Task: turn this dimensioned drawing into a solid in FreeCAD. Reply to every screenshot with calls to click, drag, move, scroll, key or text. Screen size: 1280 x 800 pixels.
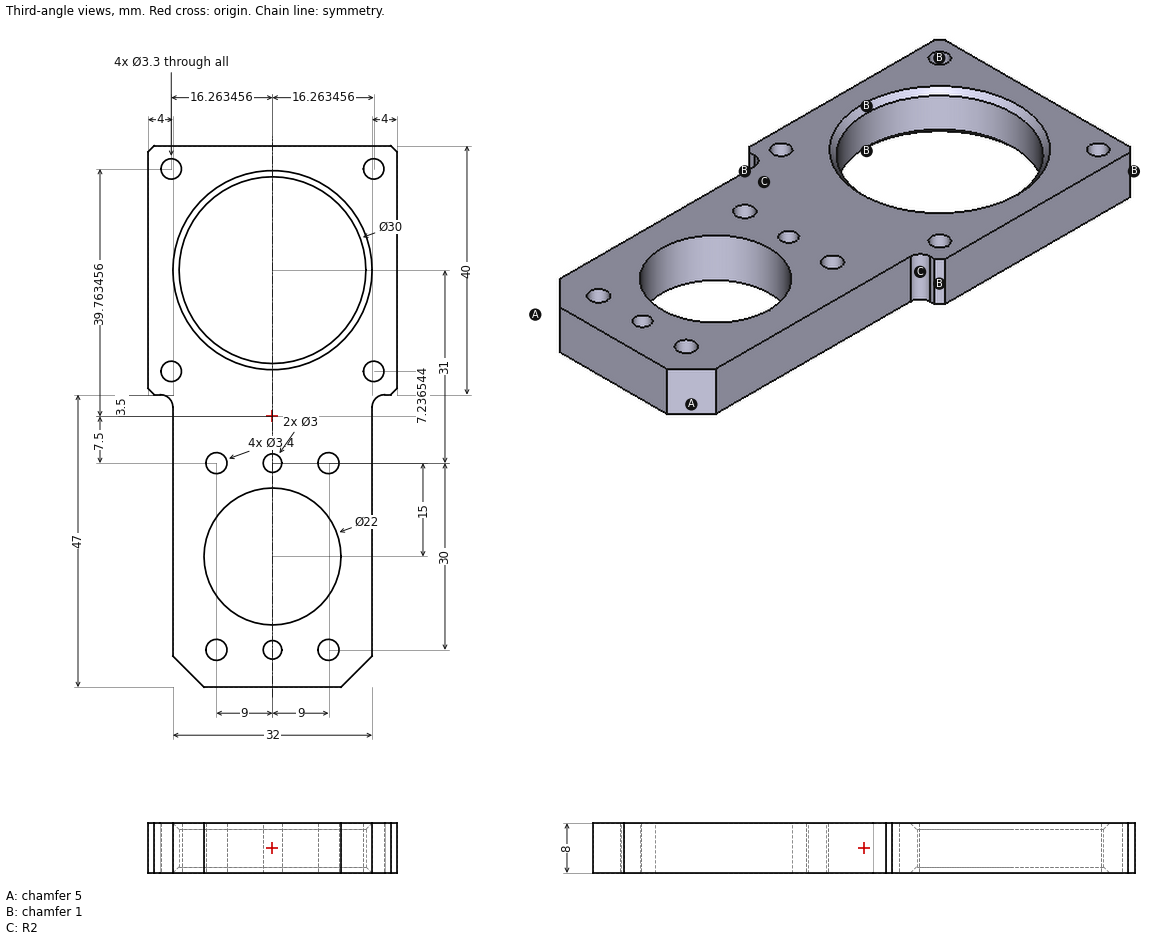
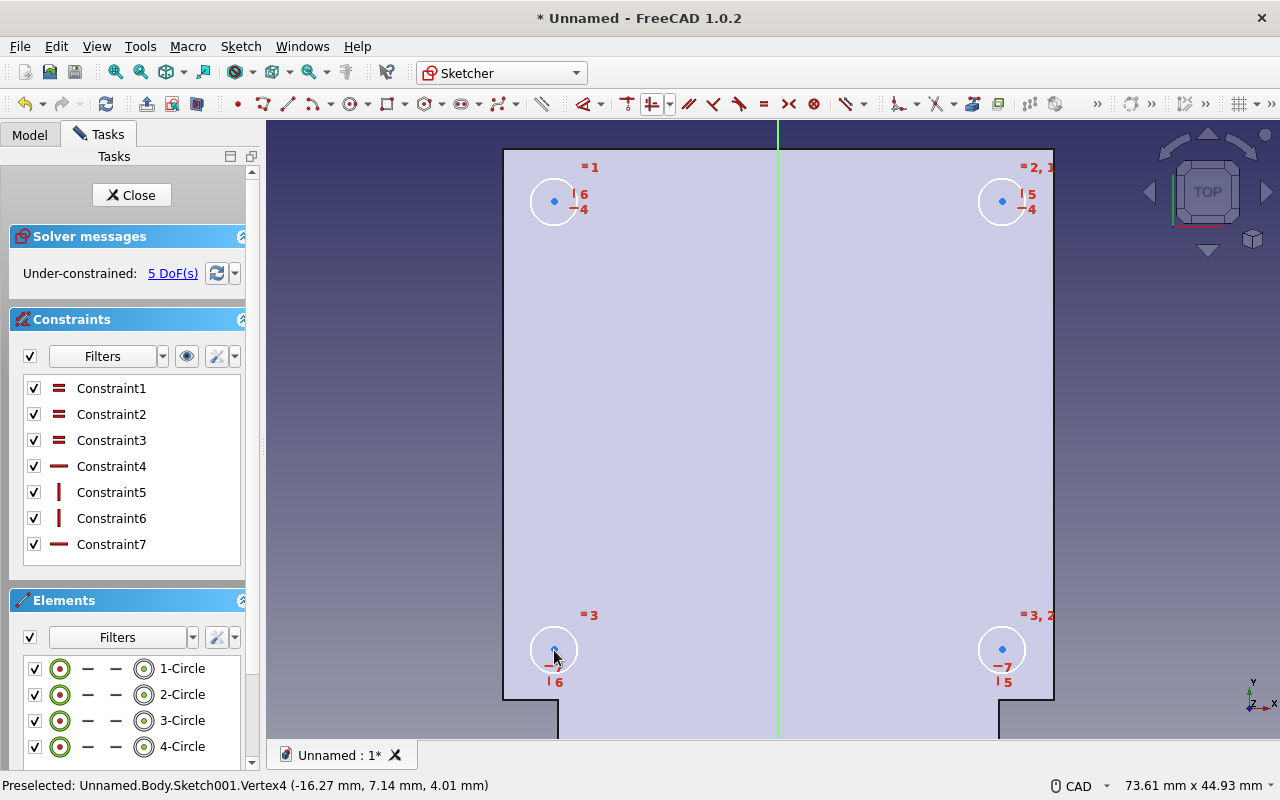
click(582, 104)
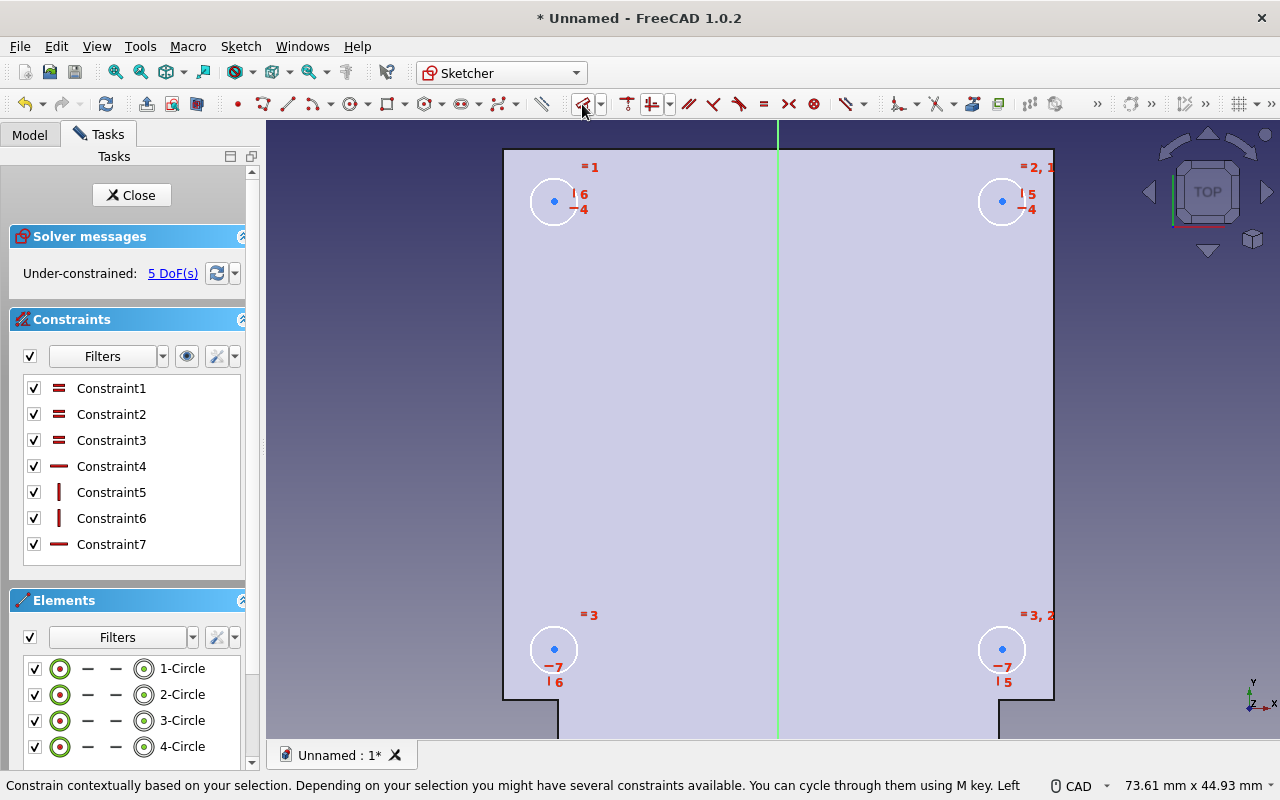
click(570, 185)
click(592, 162)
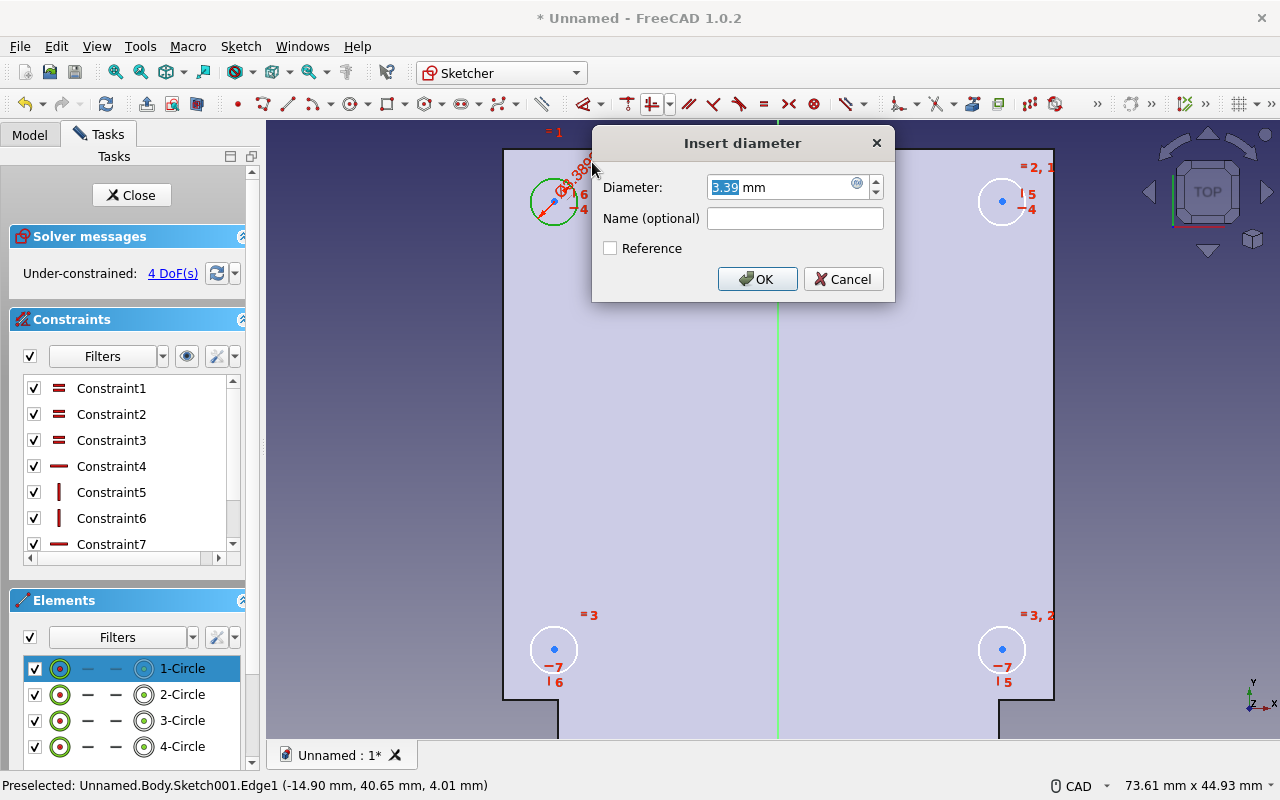
text(3.3)
key(Return)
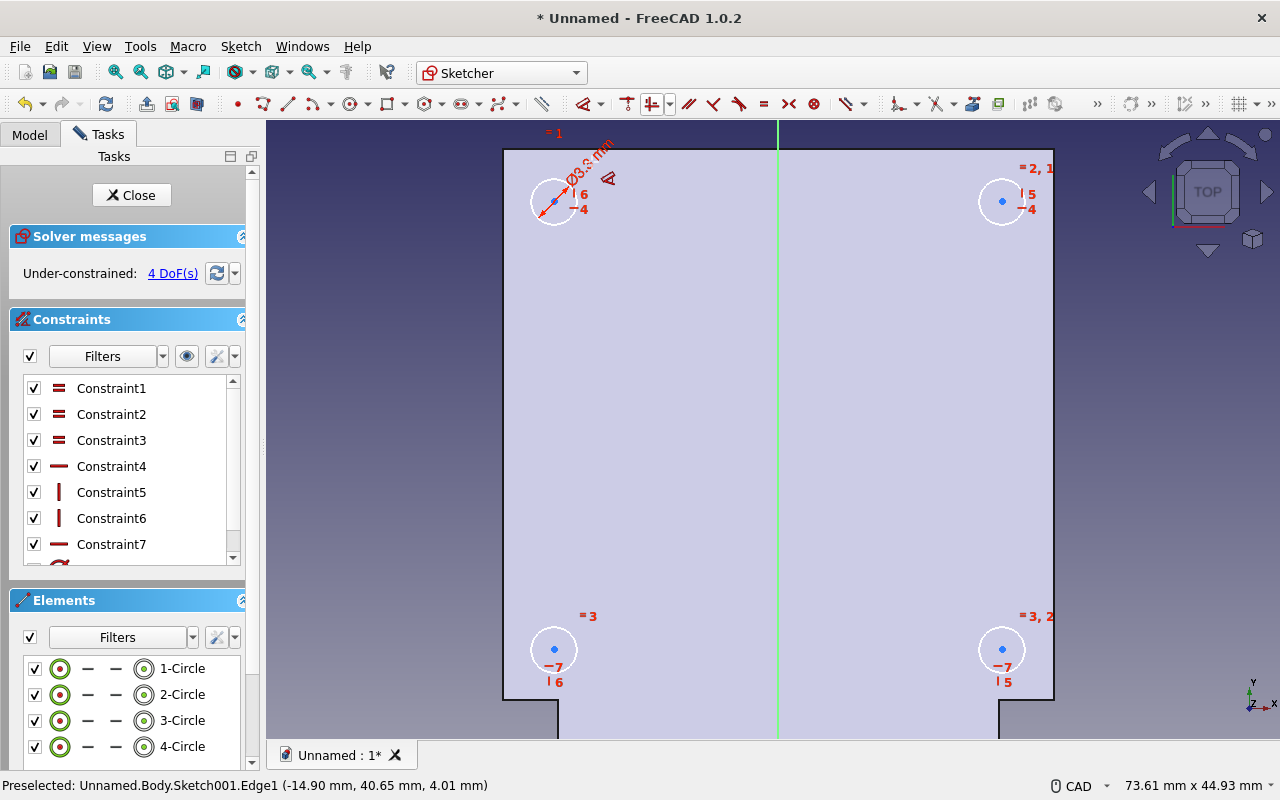
click(1002, 650)
click(1036, 680)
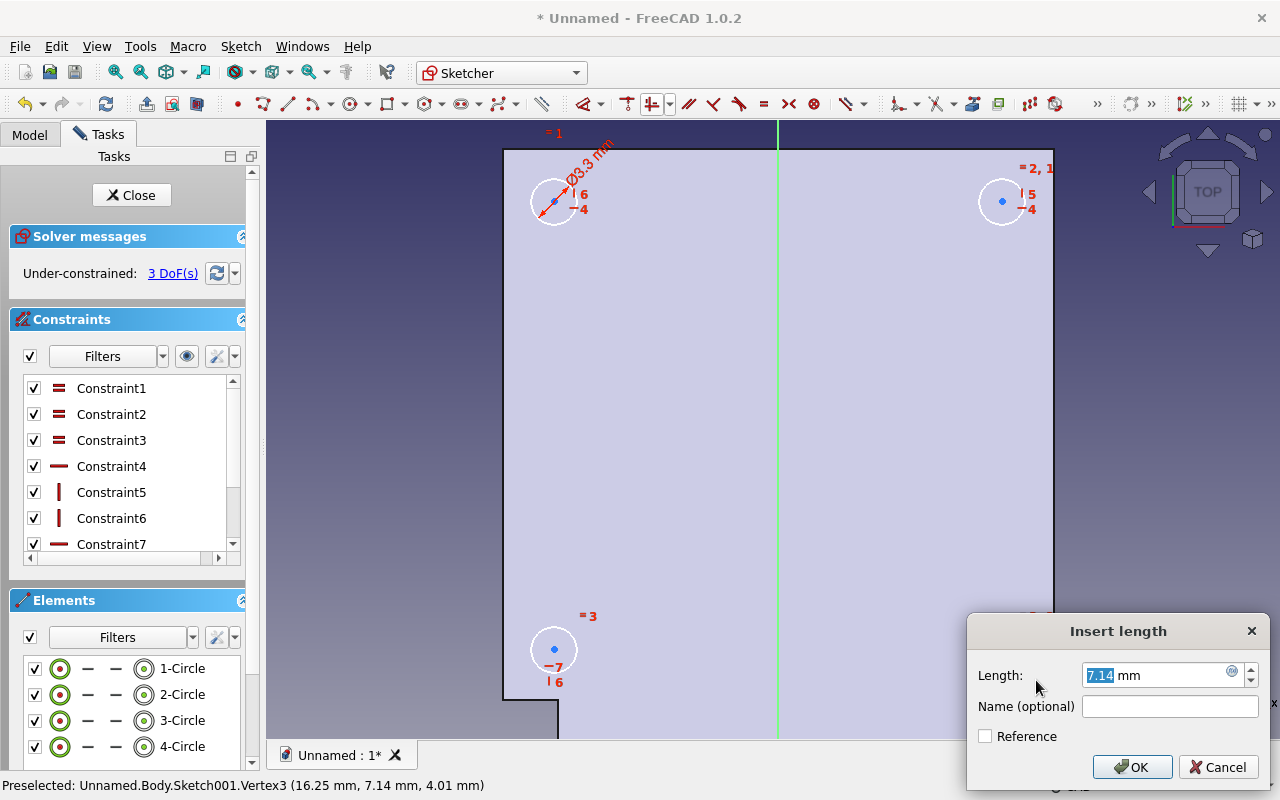
text(7.236544)
key(Return)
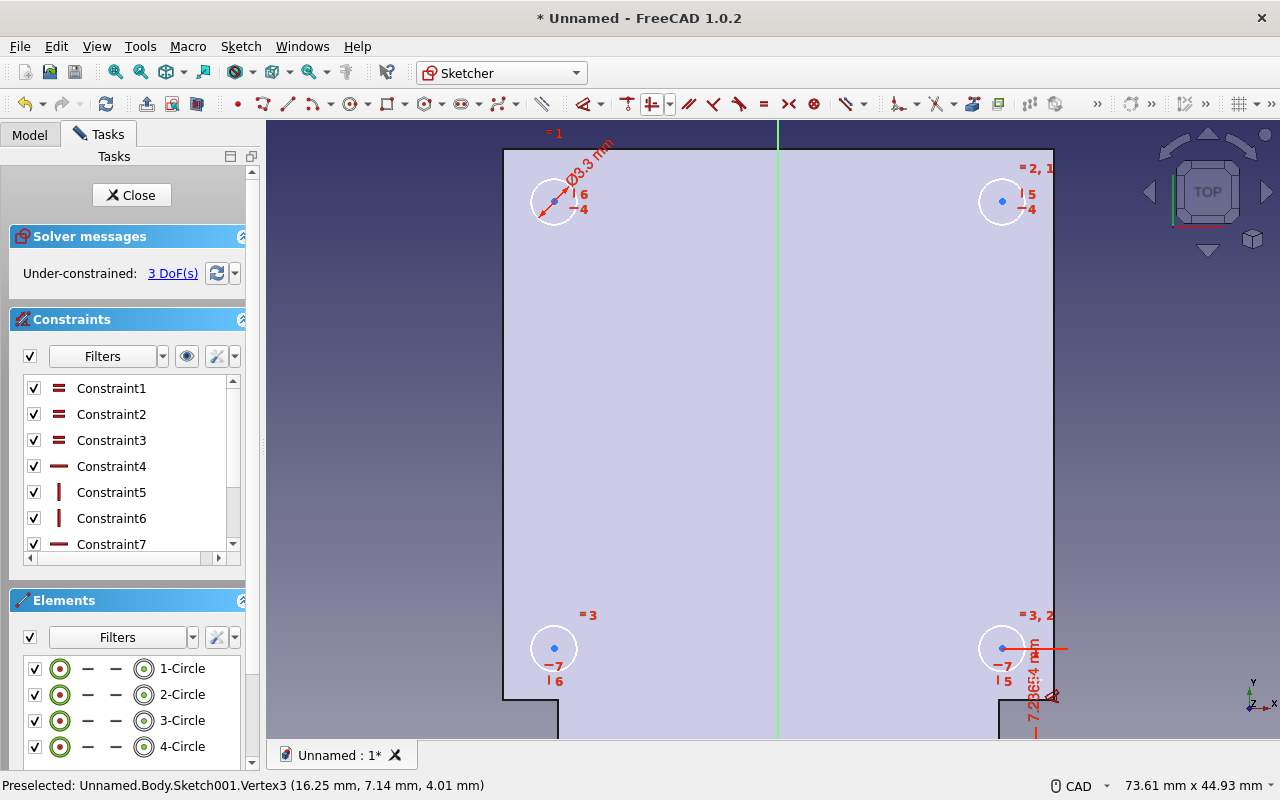
click(554, 202)
click(666, 168)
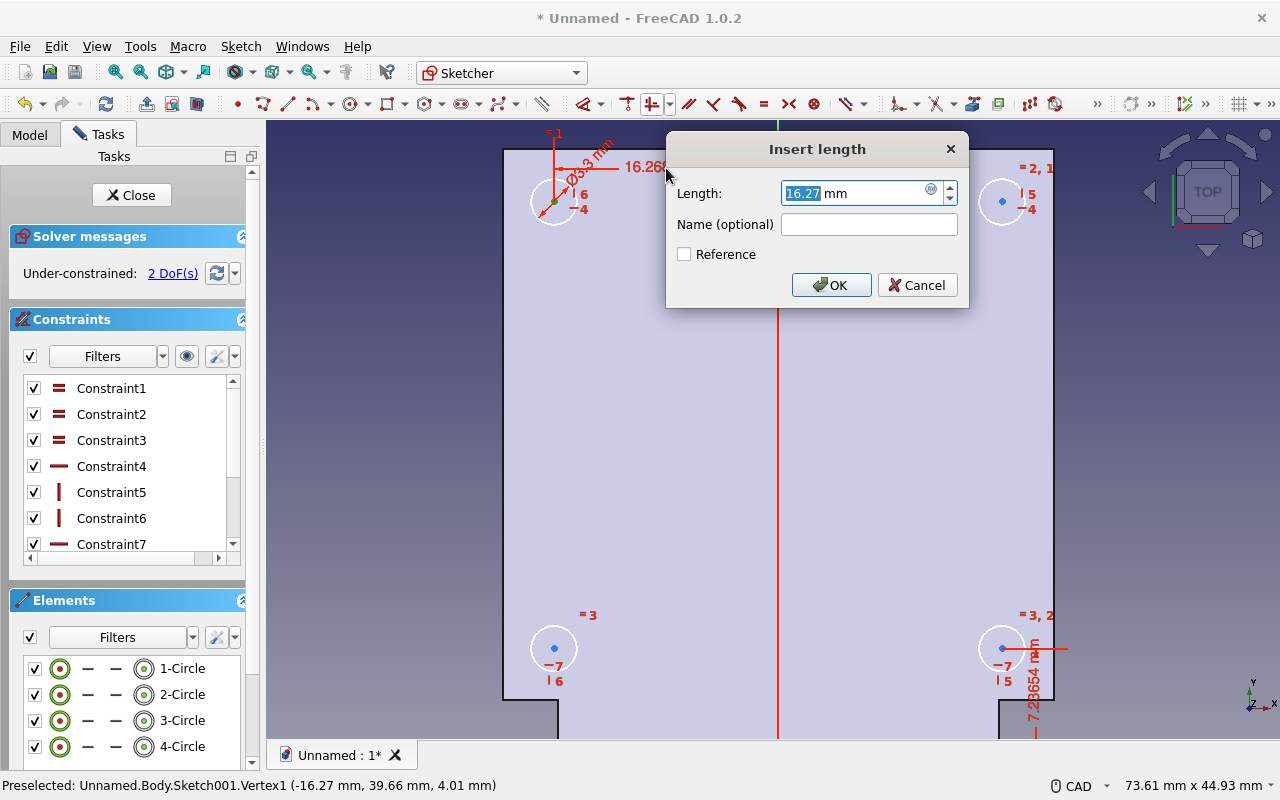
text(16.263456)
key(Return)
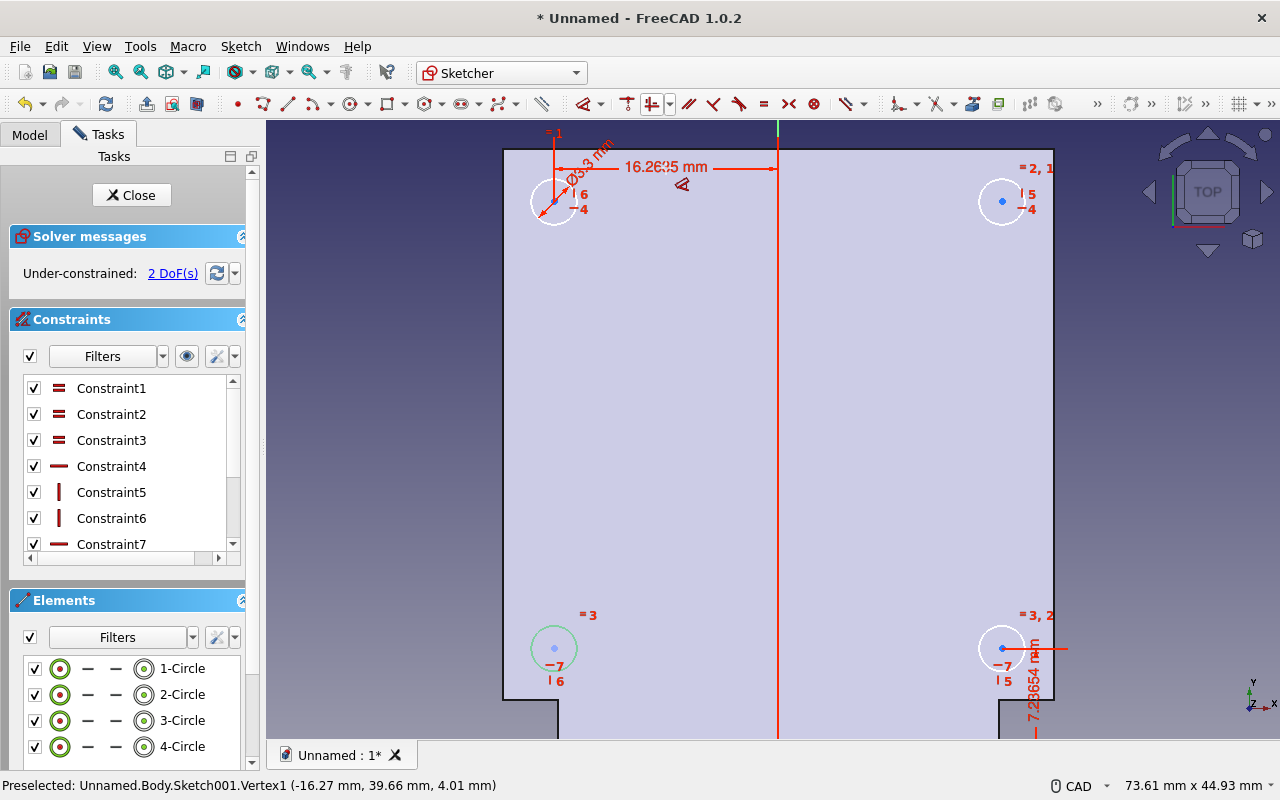
click(554, 202)
click(520, 456)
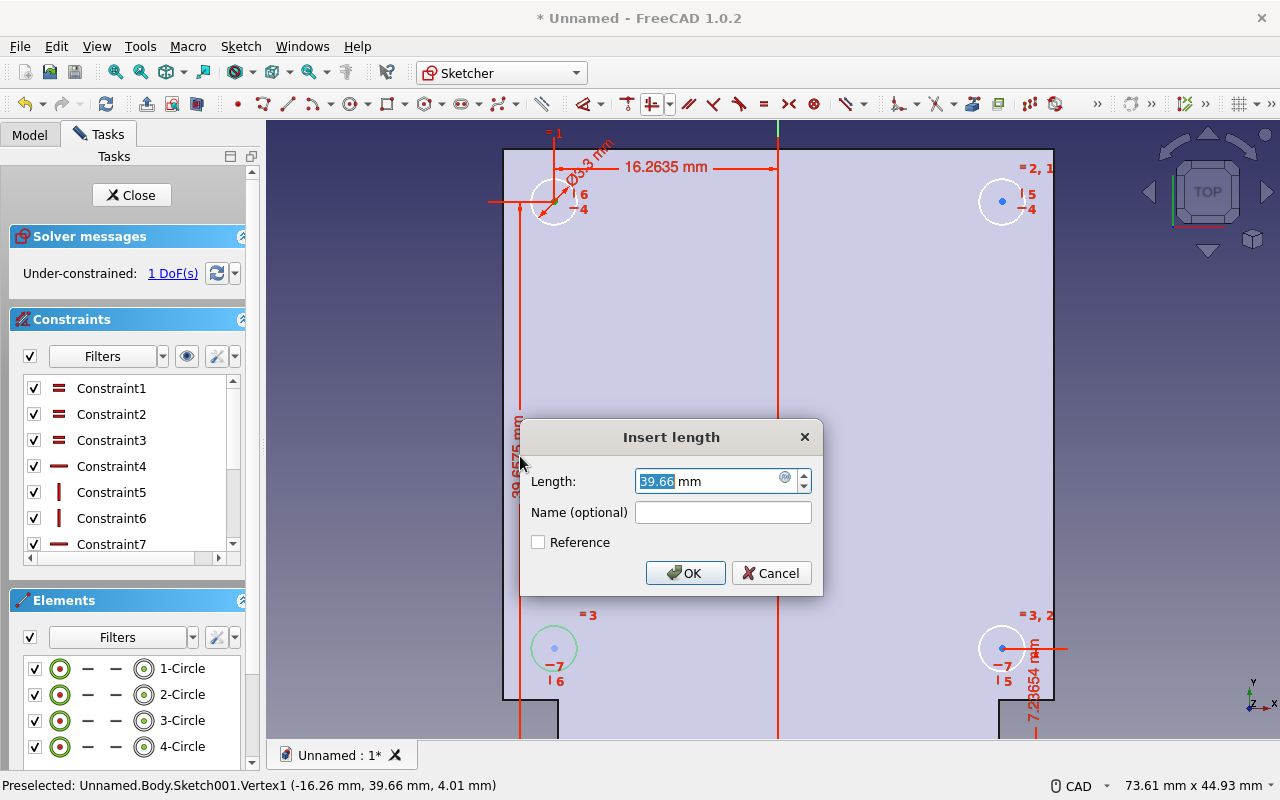
text(39.763456)
key(Return)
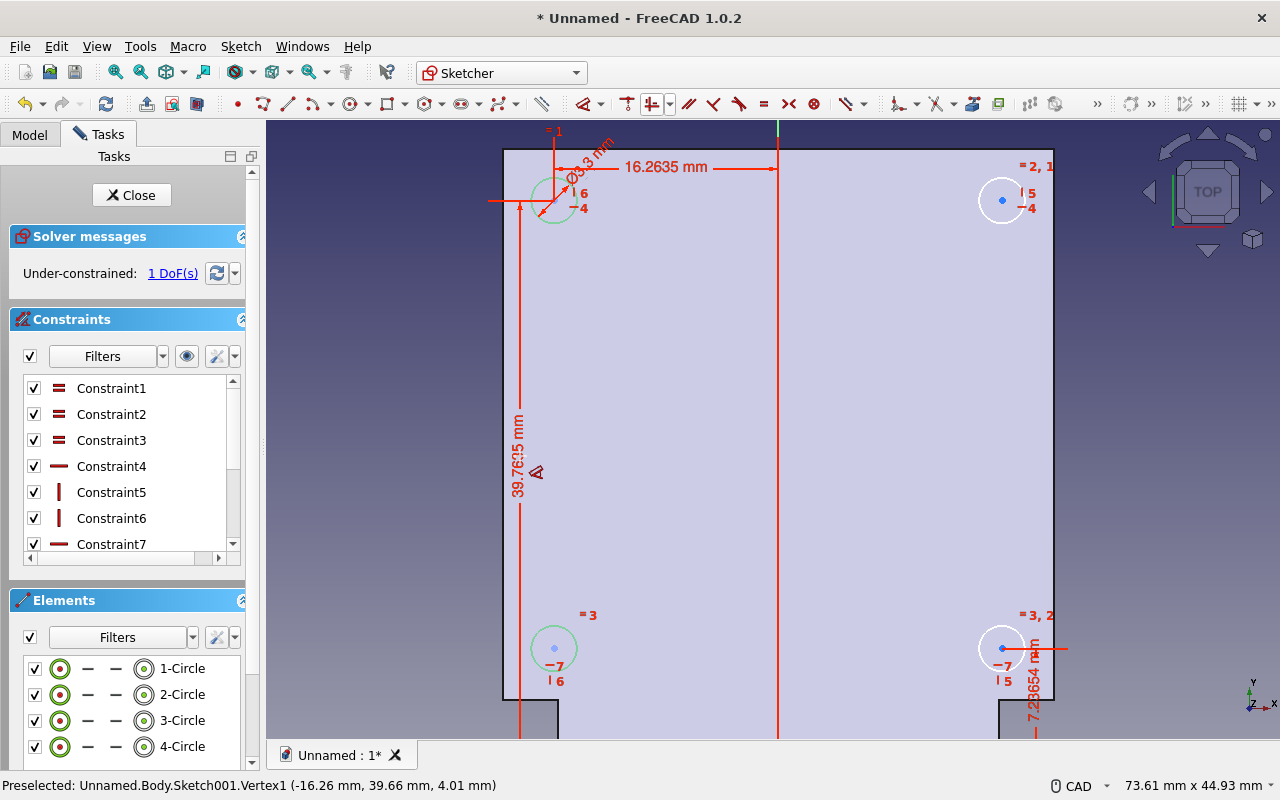
click(1002, 201)
click(890, 167)